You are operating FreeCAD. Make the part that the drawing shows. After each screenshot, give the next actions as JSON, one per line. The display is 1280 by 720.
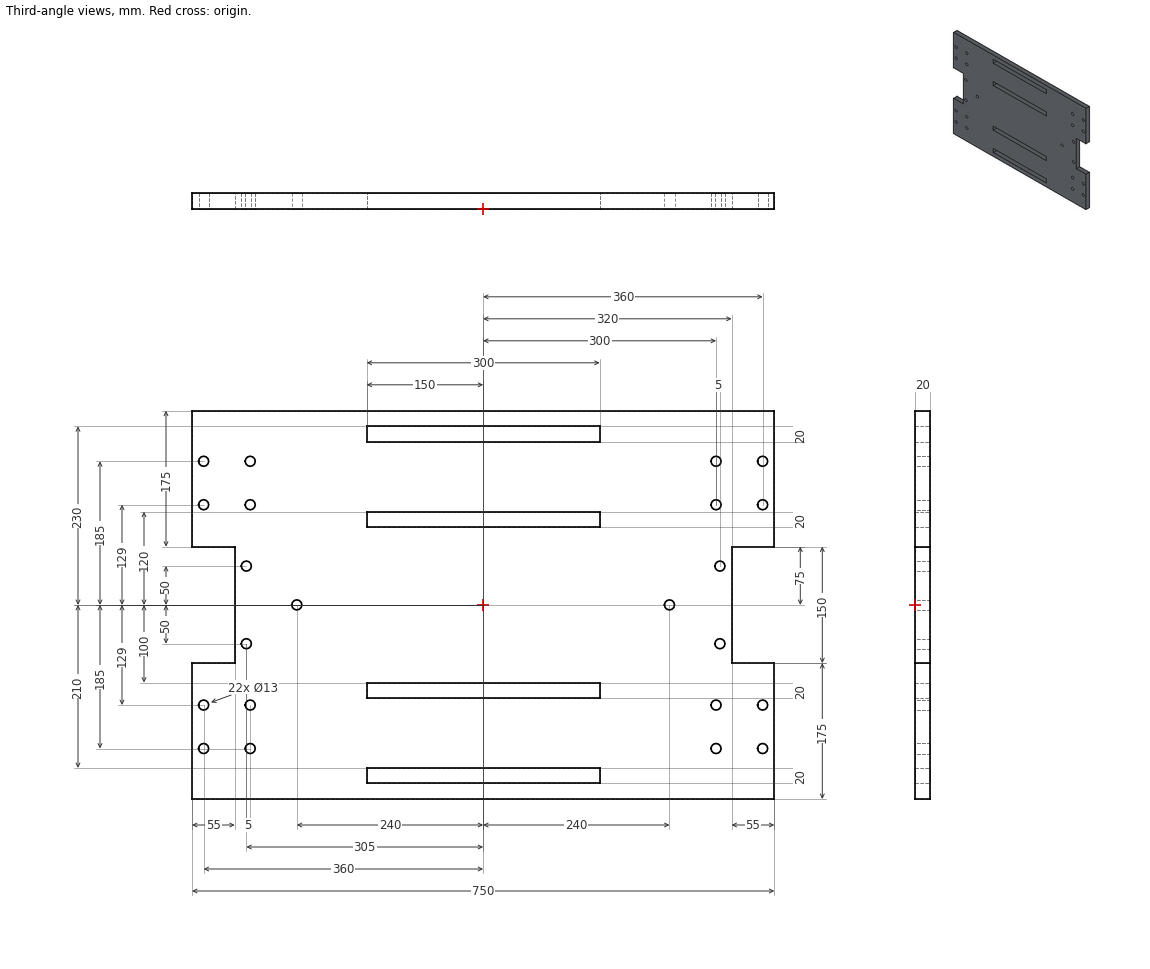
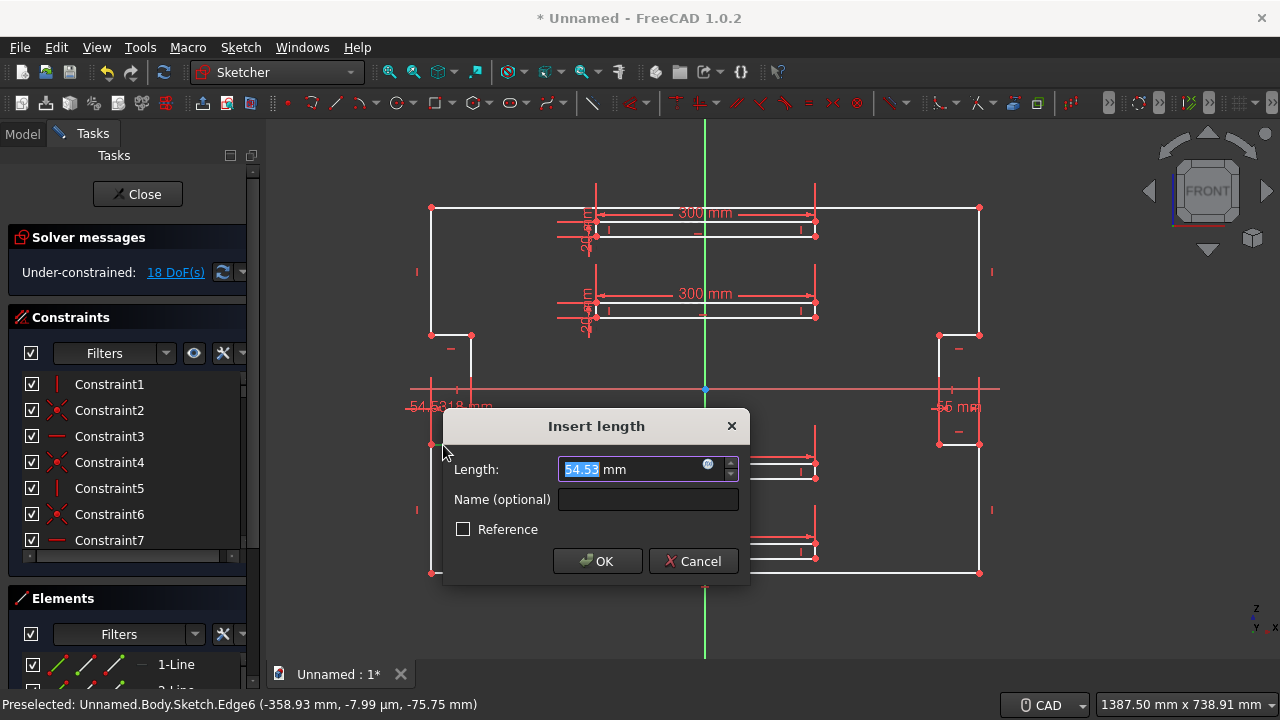
{"action": "type", "text": "55"}
{"action": "key", "text": "Return"}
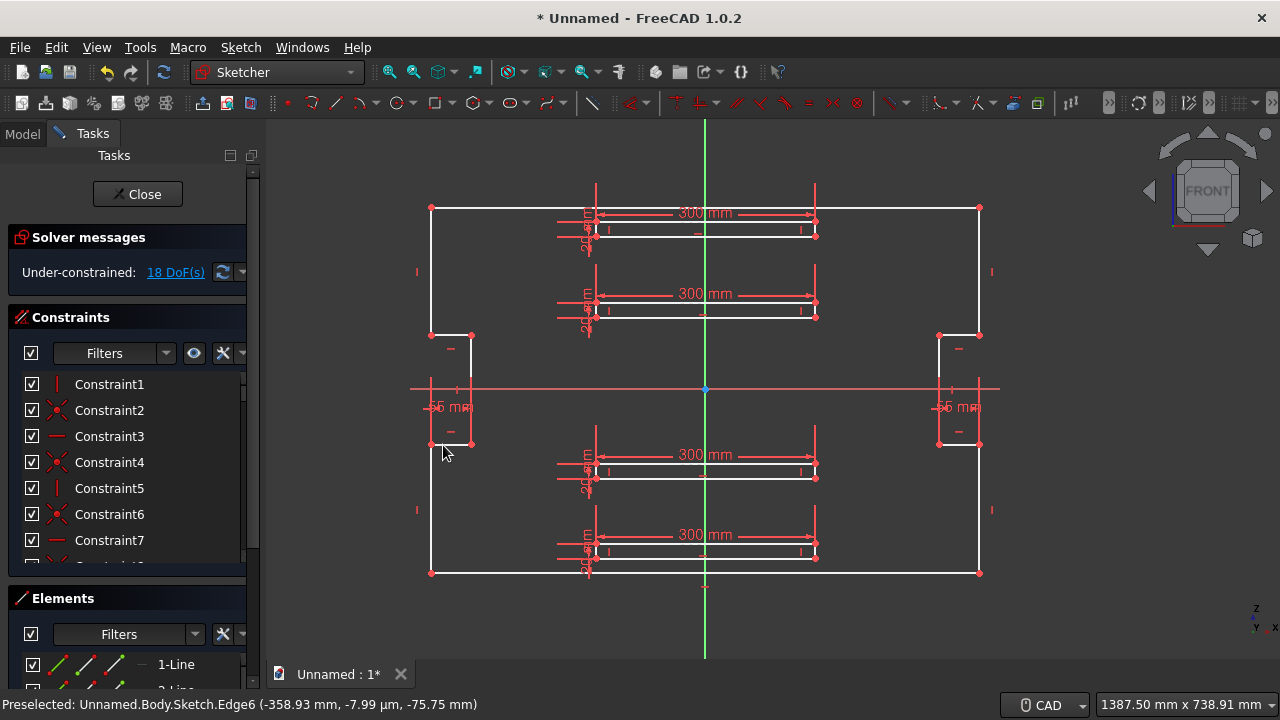
{"action": "left_click", "coordinate": [459, 335]}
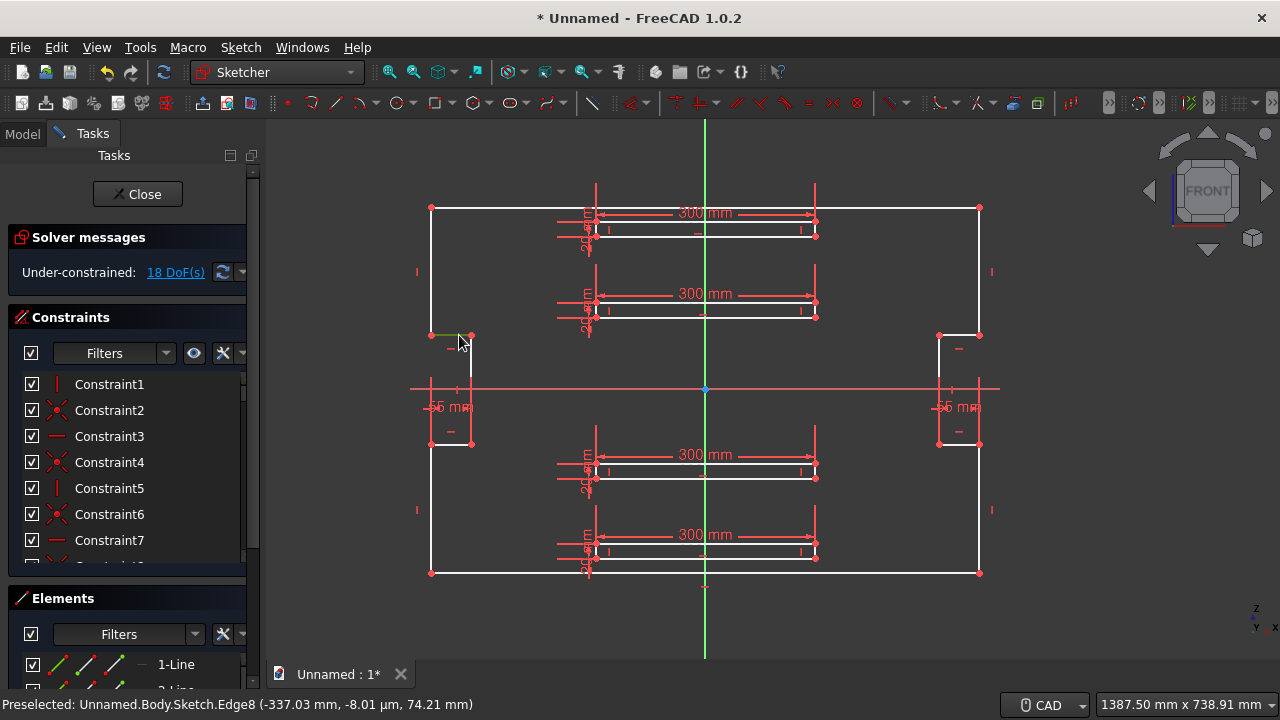
{"action": "key", "text": "l"}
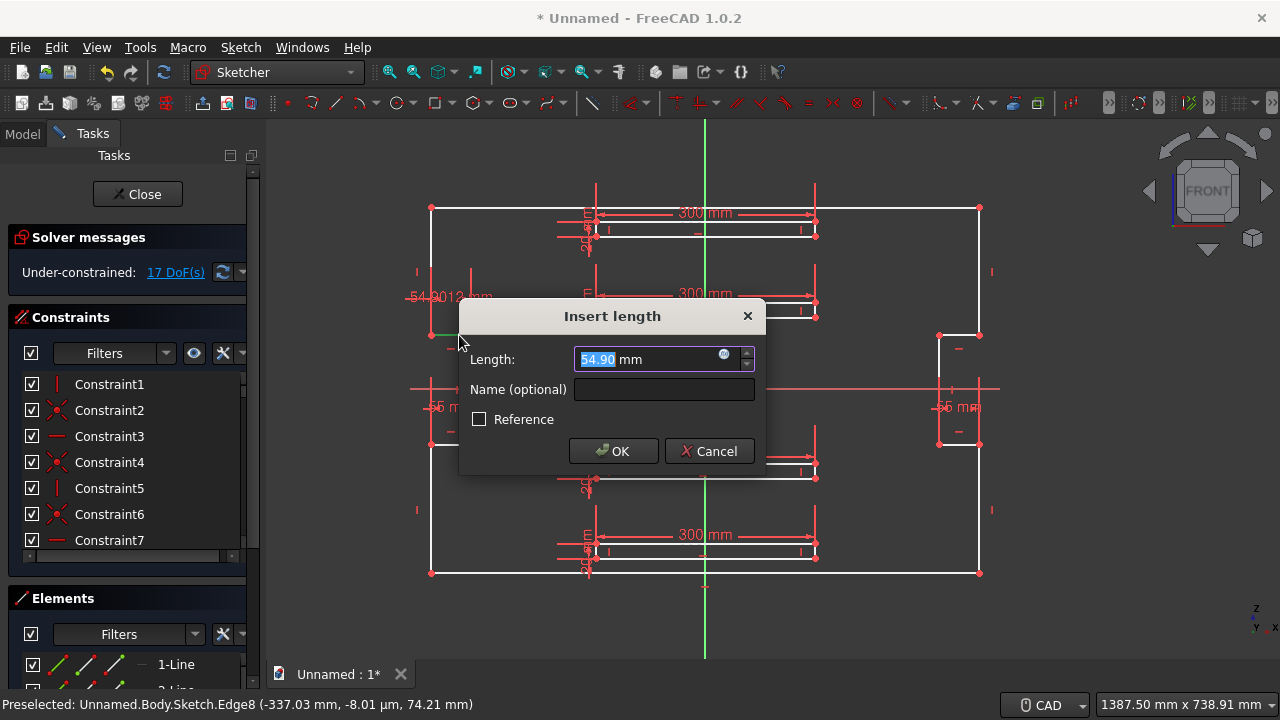
{"action": "type", "text": "55"}
{"action": "key", "text": "Return"}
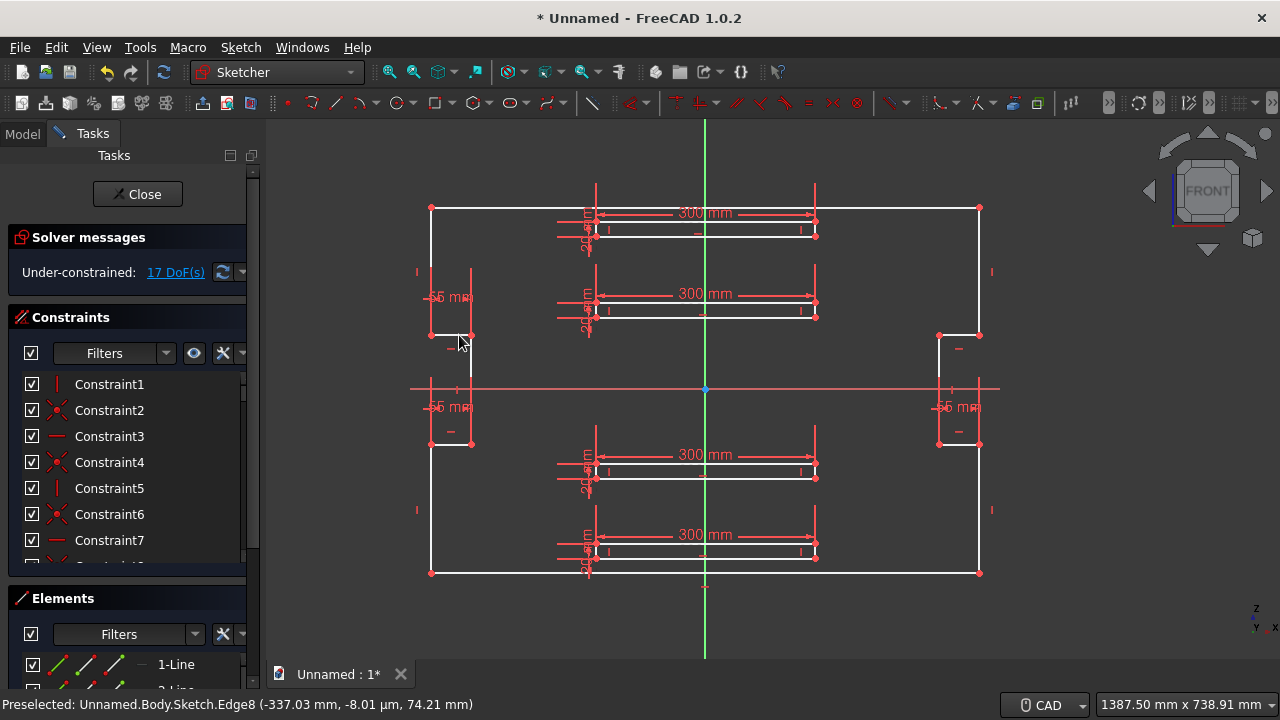
{"action": "left_click", "coordinate": [967, 335]}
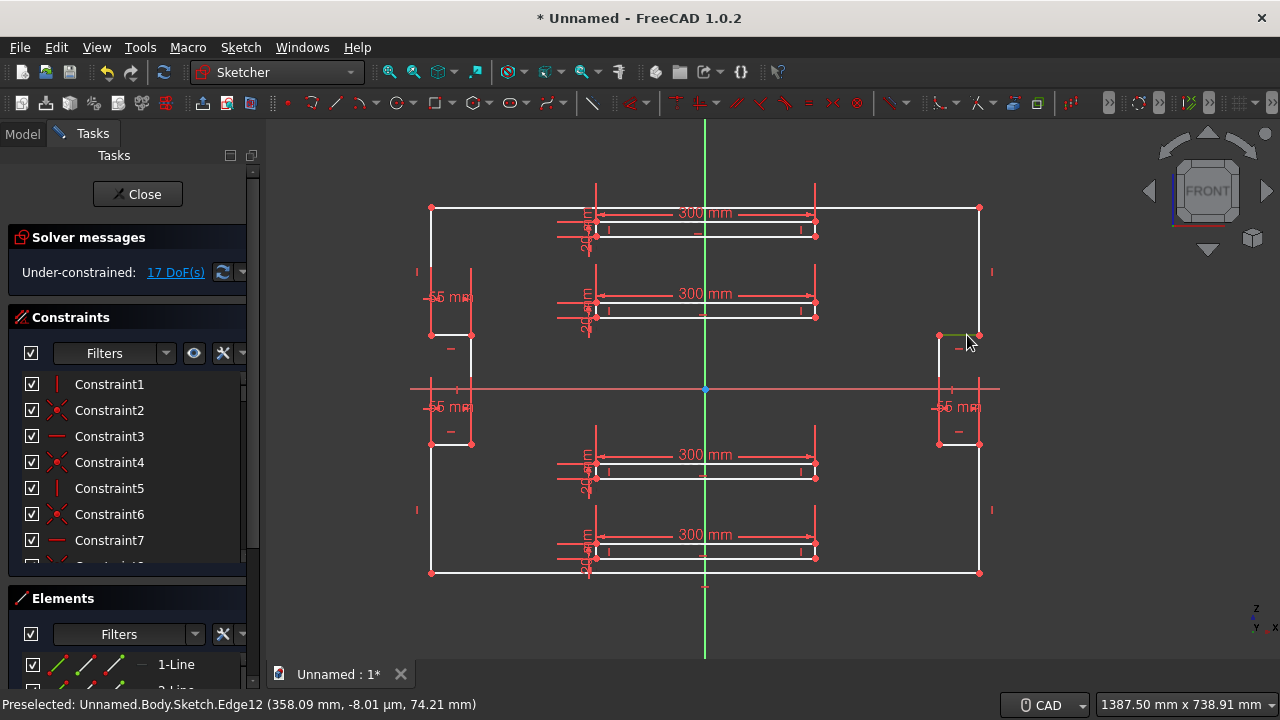
{"action": "left_click", "coordinate": [648, 104]}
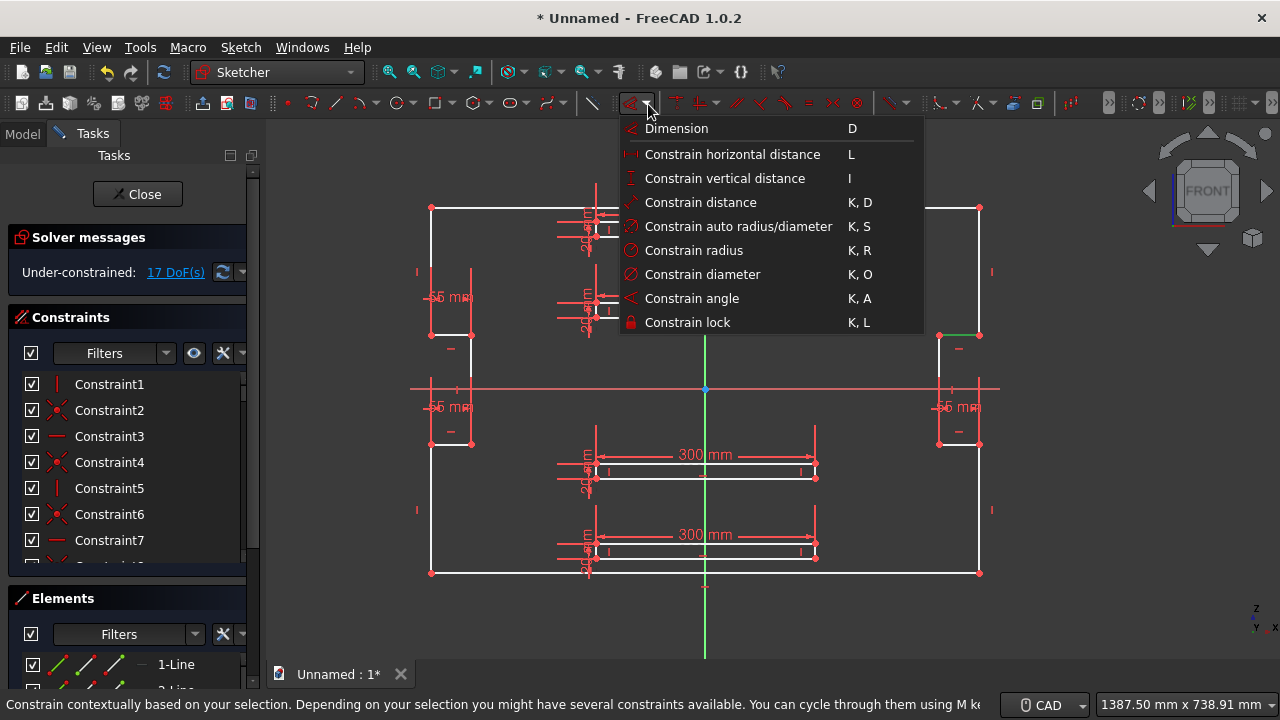
{"action": "left_click", "coordinate": [772, 154]}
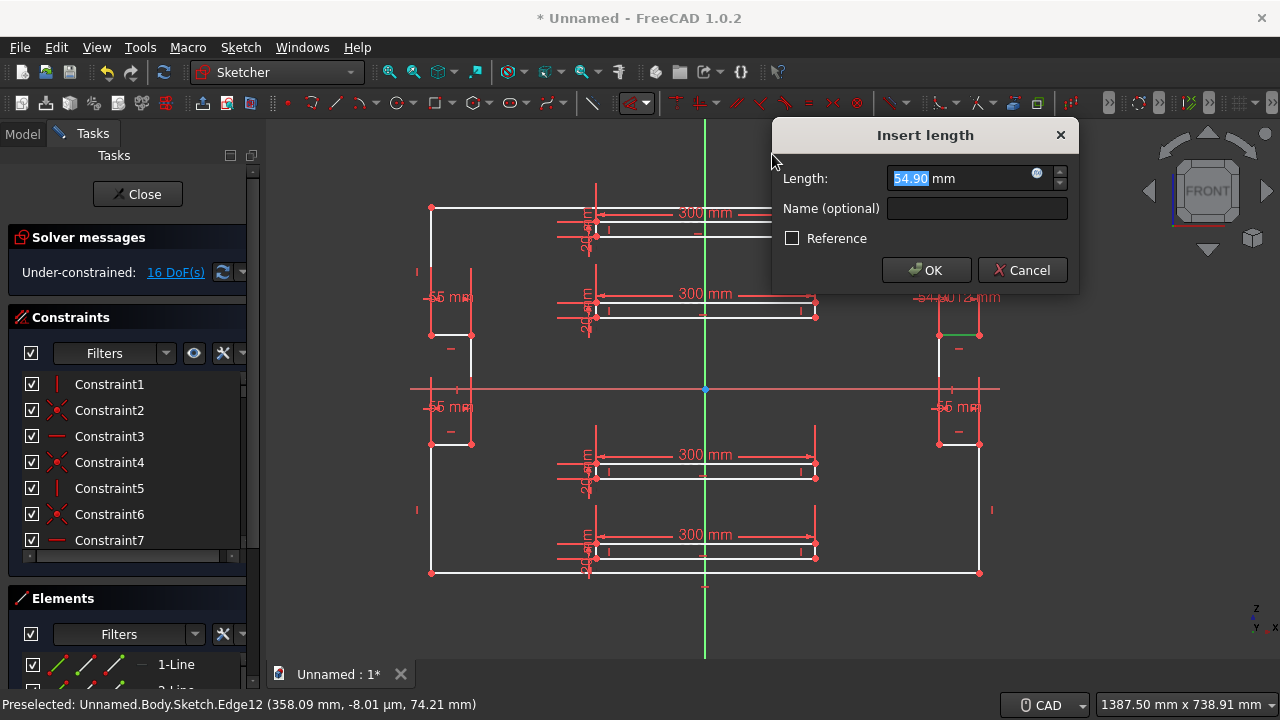
{"action": "type", "text": "55"}
{"action": "key", "text": "Return"}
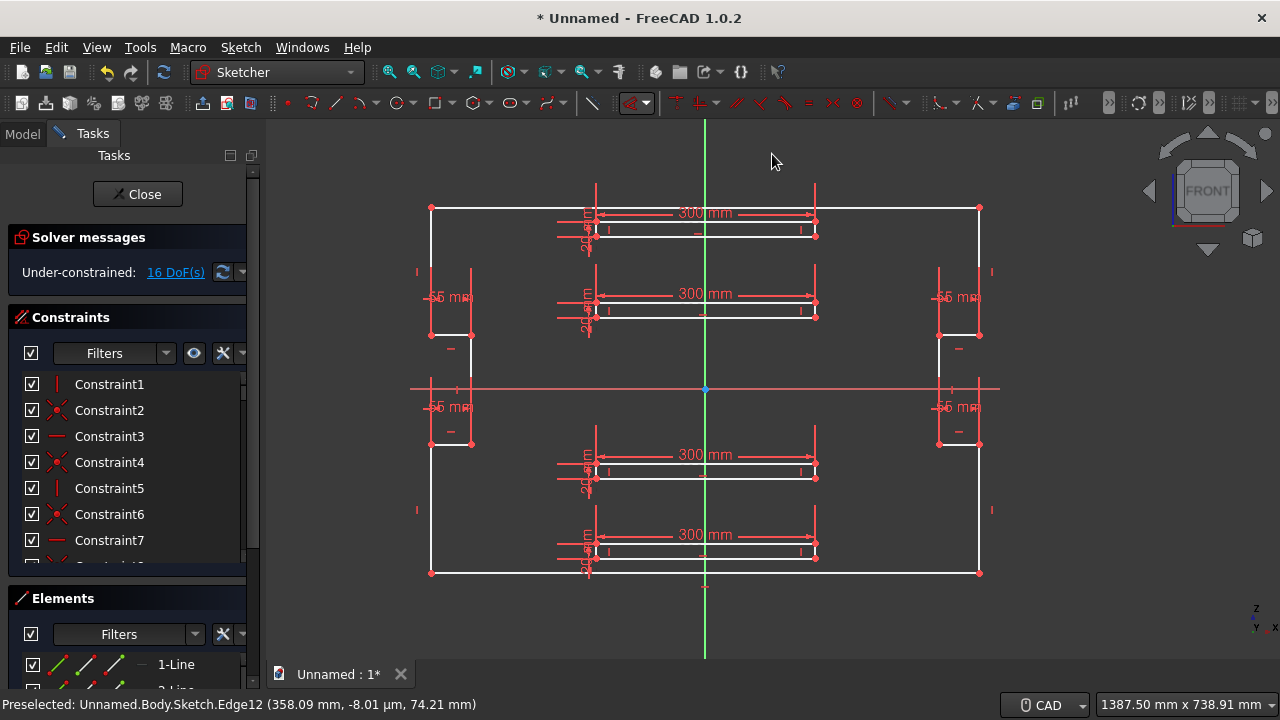
{"action": "left_click", "coordinate": [939, 368]}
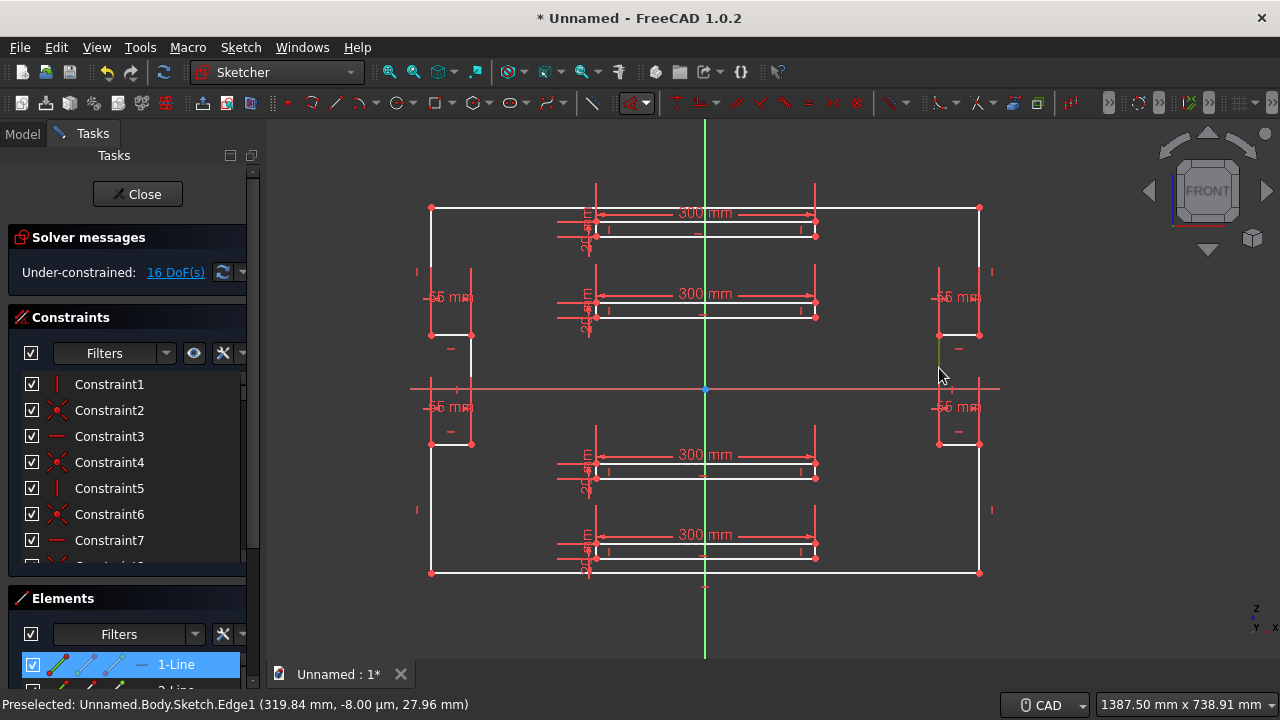
{"action": "key", "text": "i"}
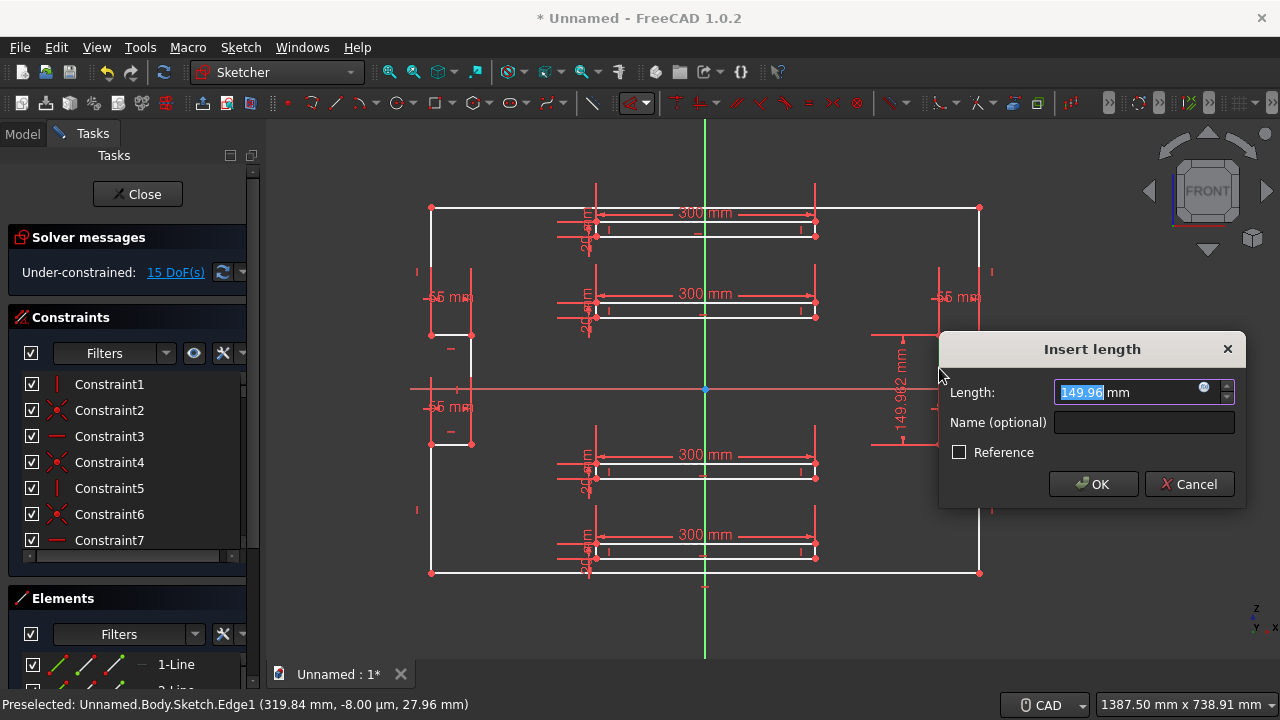
{"action": "type", "text": "150"}
{"action": "key", "text": "Return"}